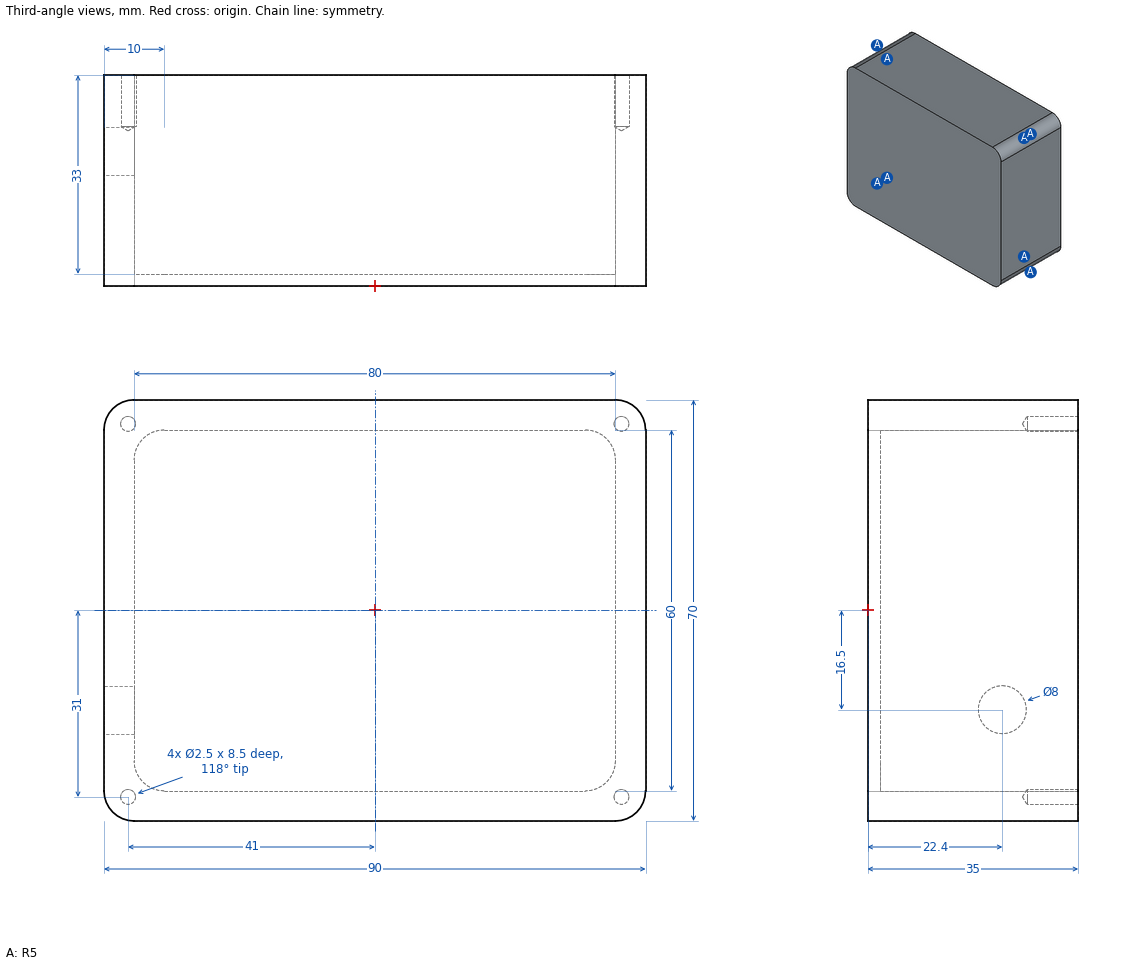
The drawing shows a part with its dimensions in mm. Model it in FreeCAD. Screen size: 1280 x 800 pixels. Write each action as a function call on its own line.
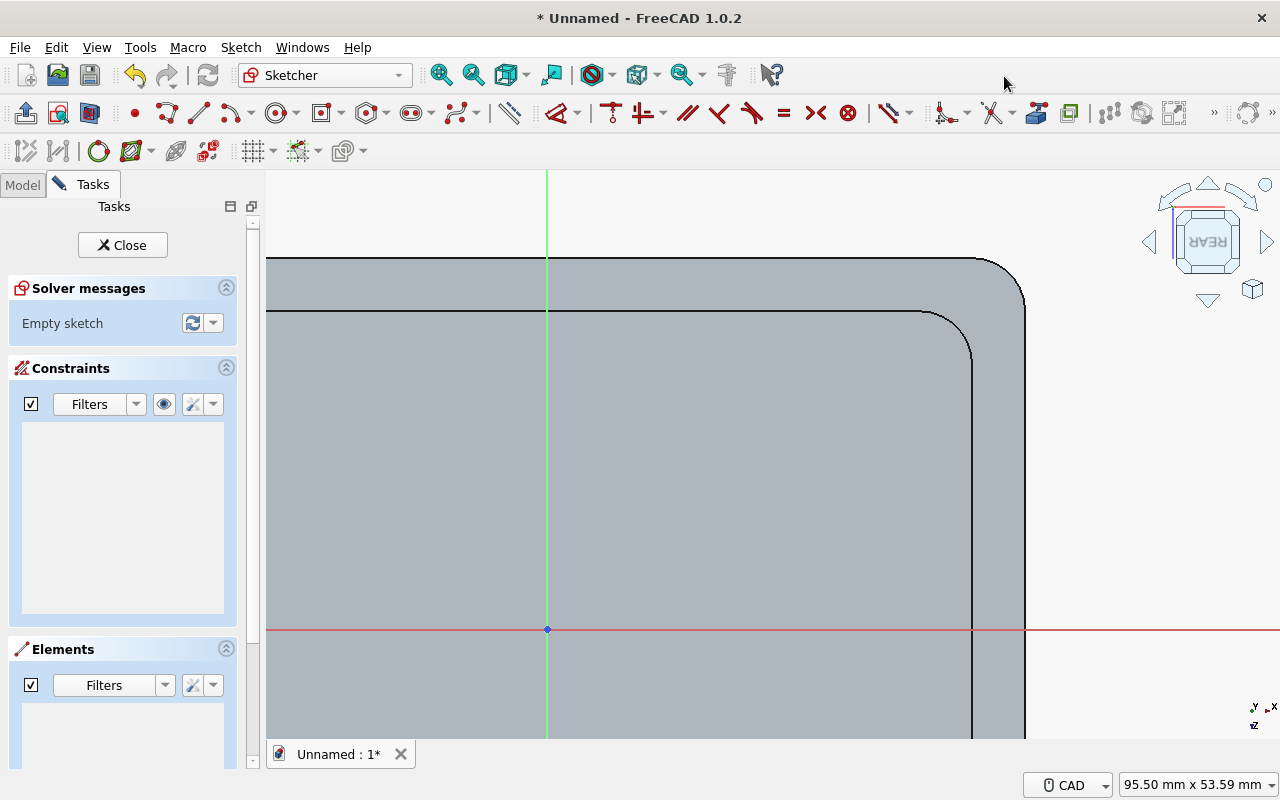
scroll(896, 241, down, 3)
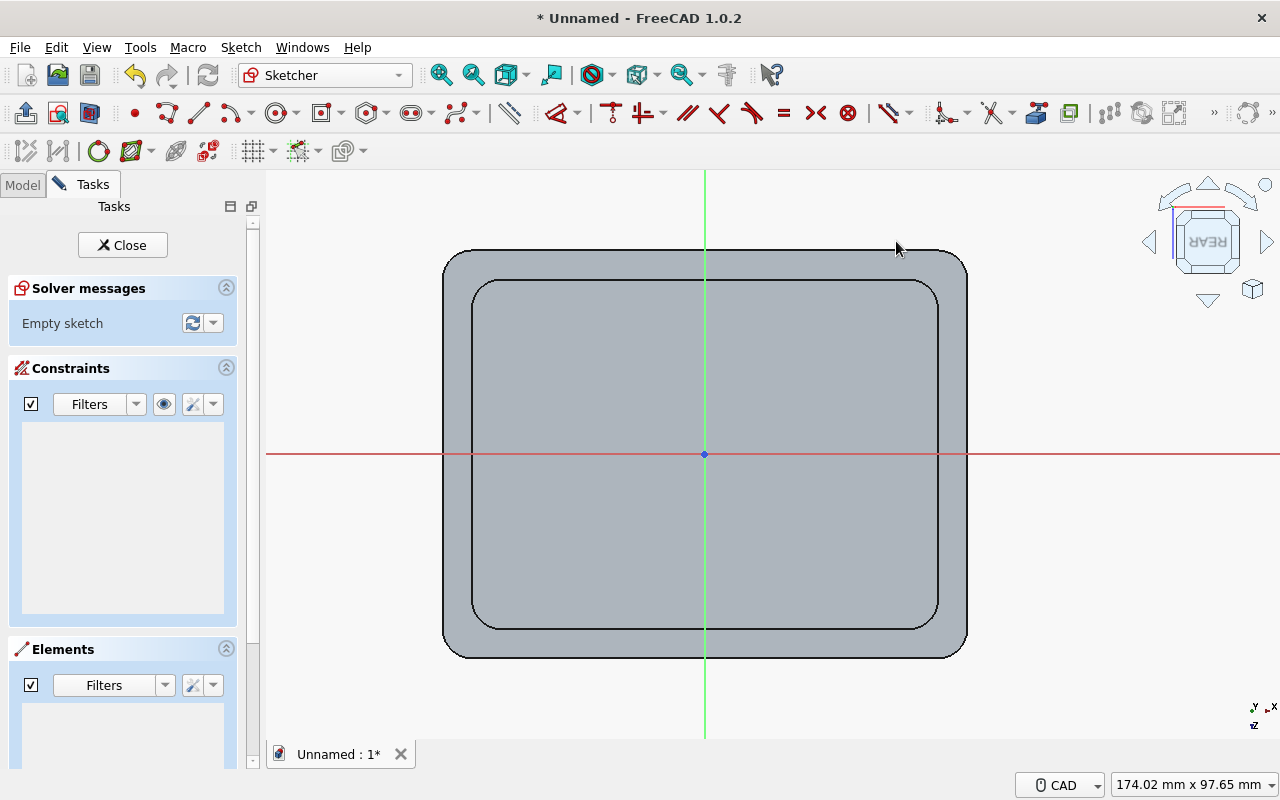
click(276, 114)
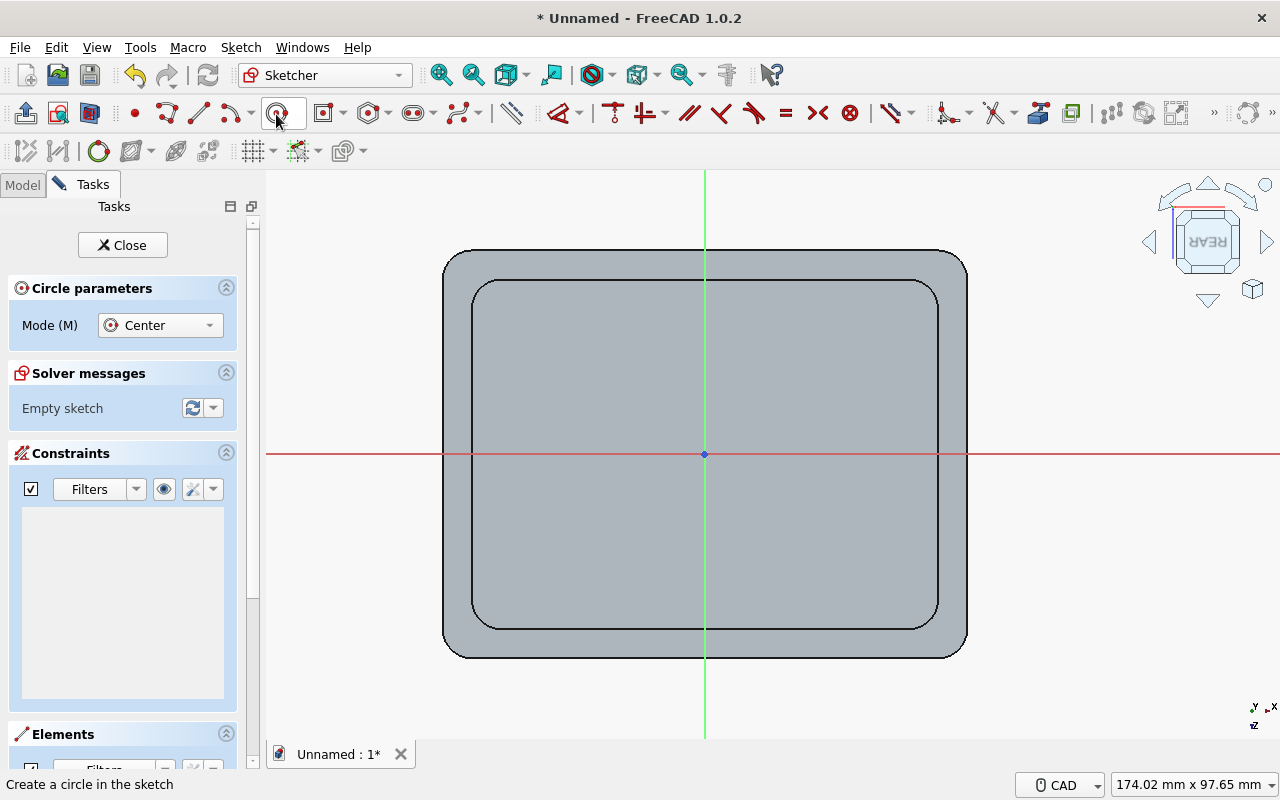
scroll(466, 274, up, 6)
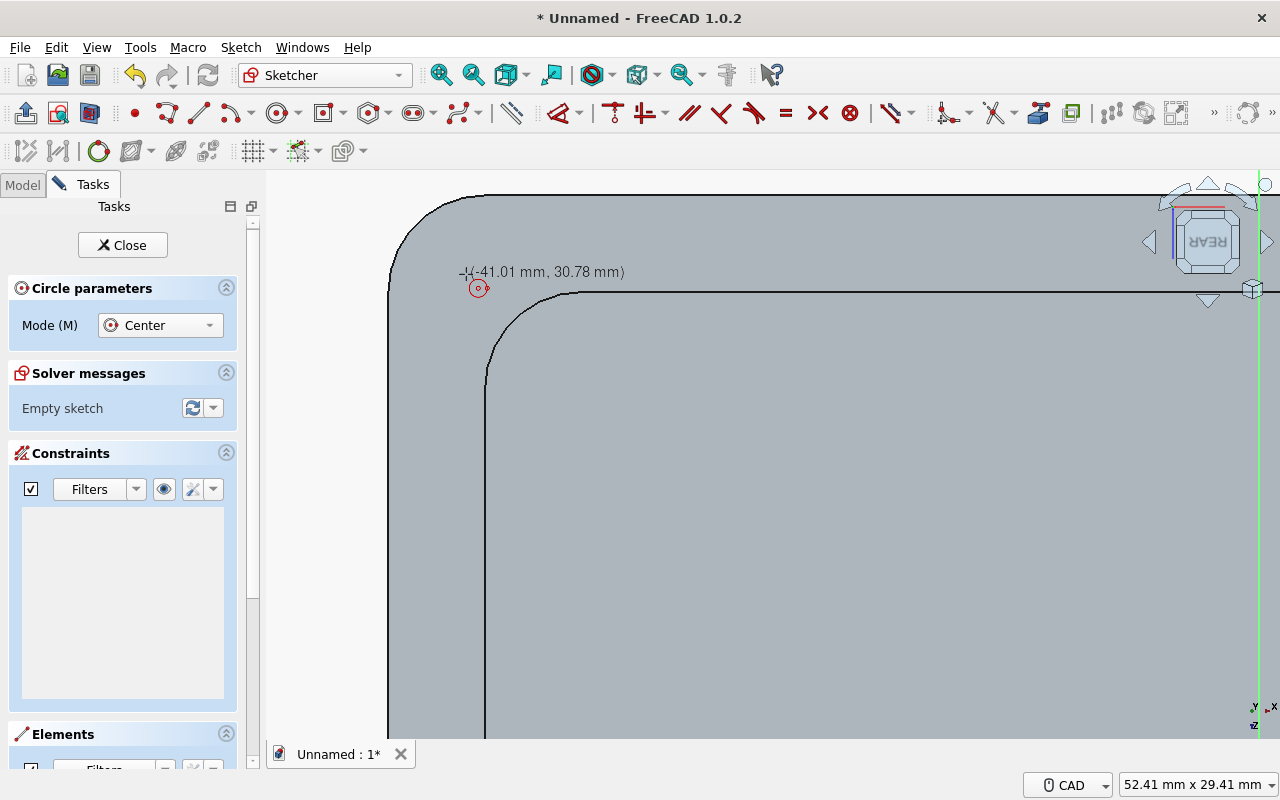
click(466, 273)
click(483, 256)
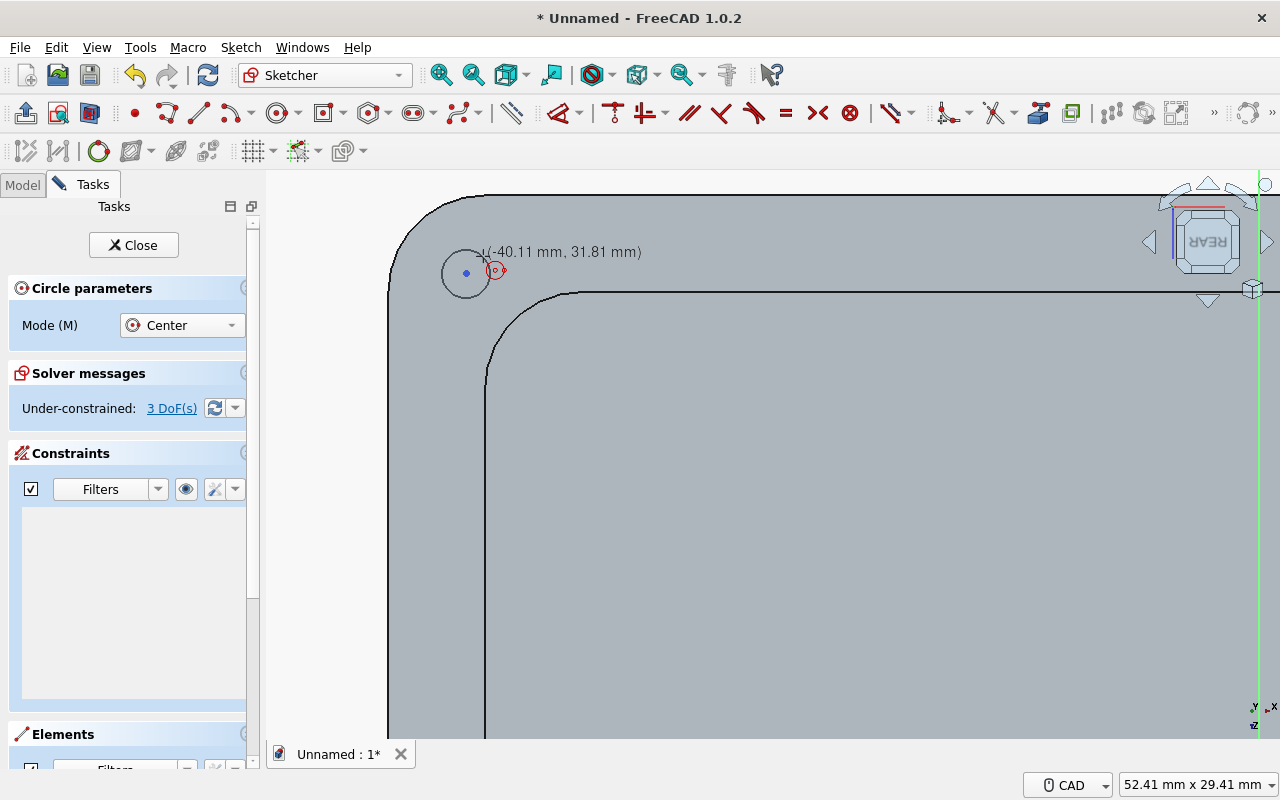
scroll(466, 274, down, 6)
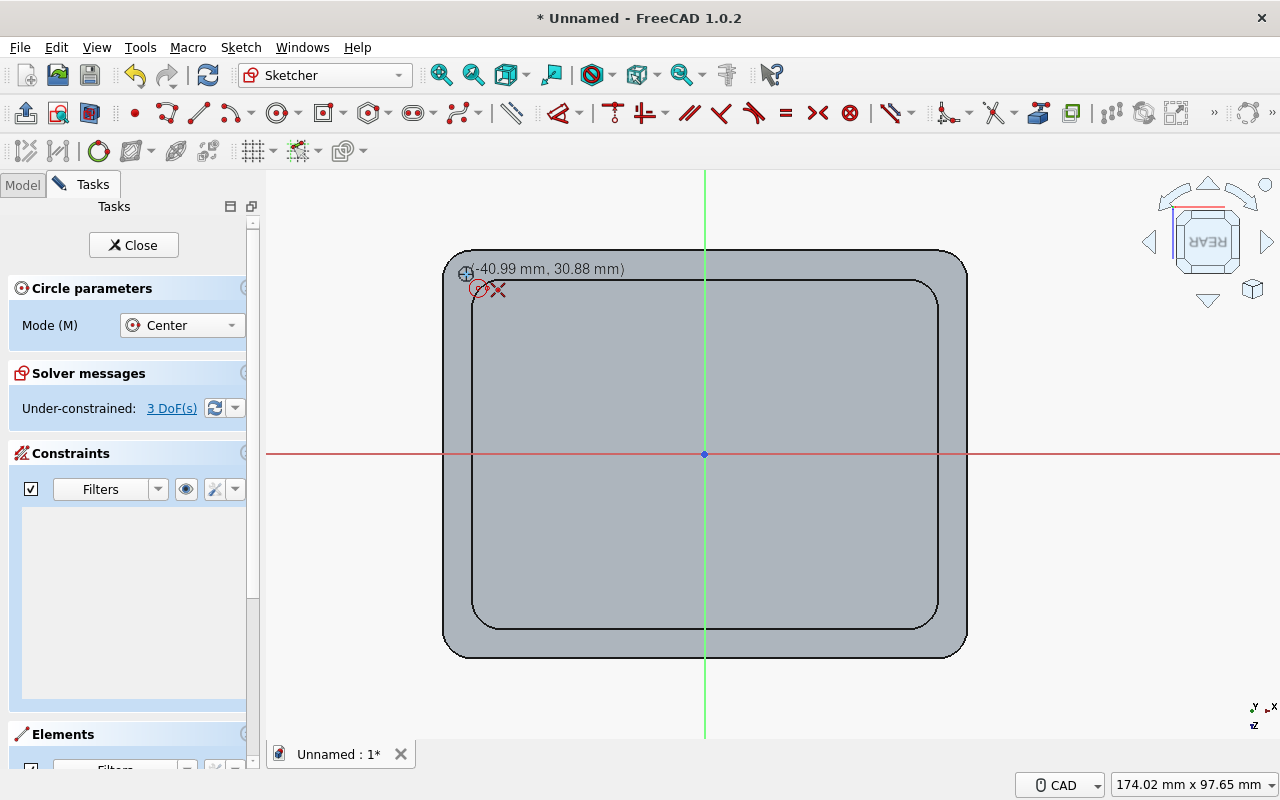
scroll(944, 274, up, 6)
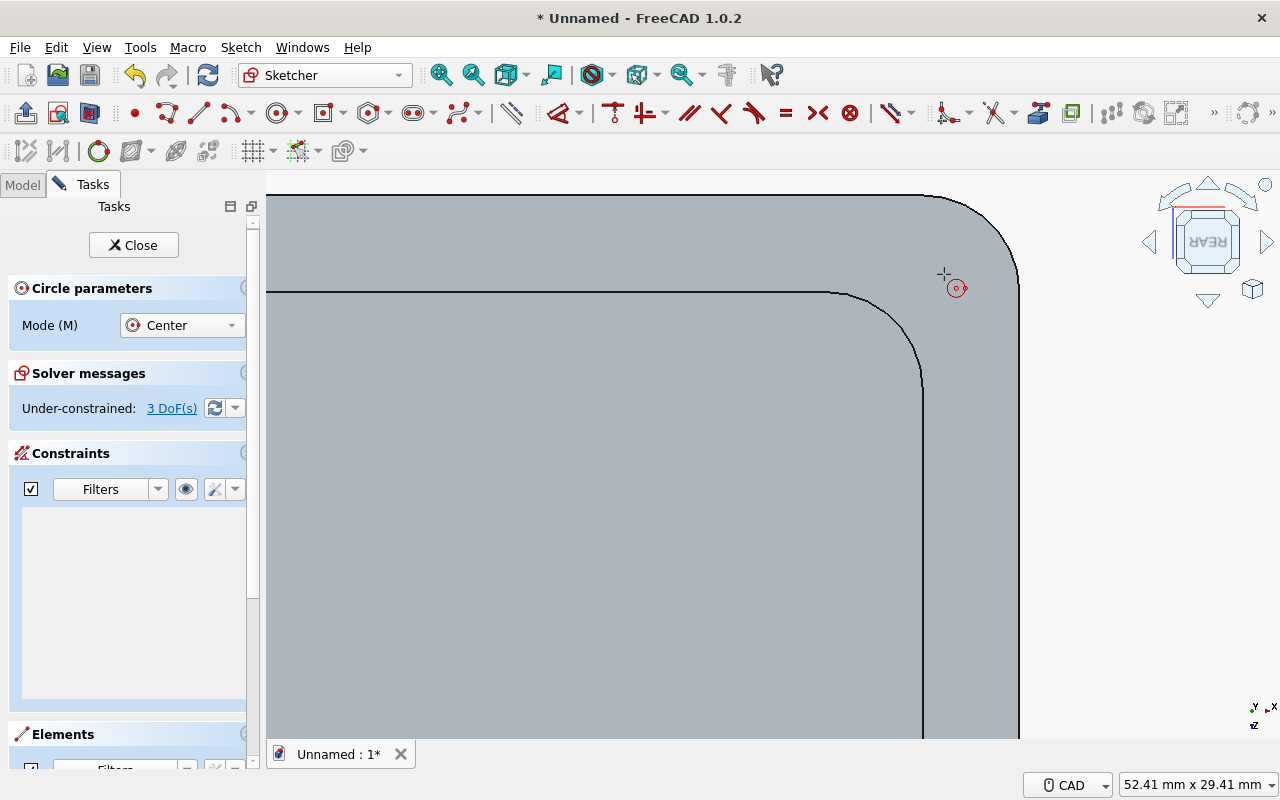
click(942, 273)
click(959, 256)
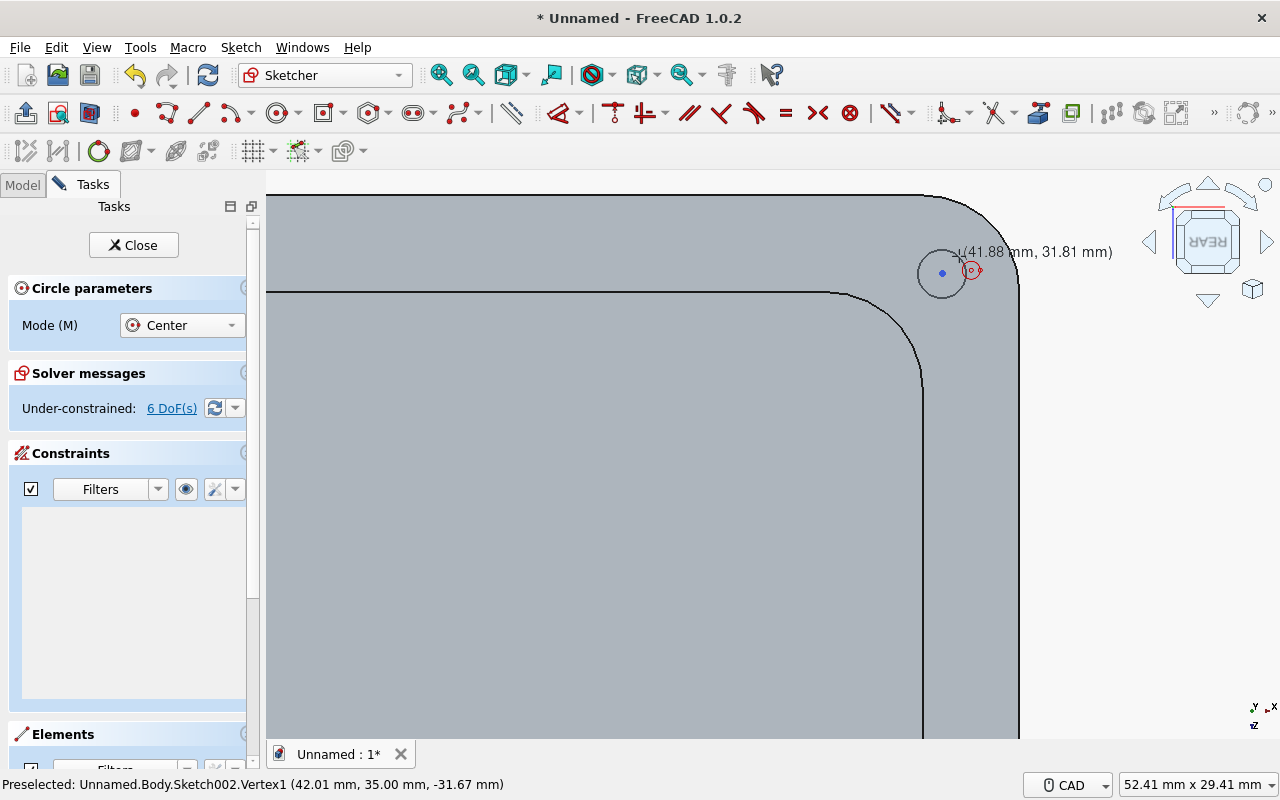
scroll(944, 274, down, 6)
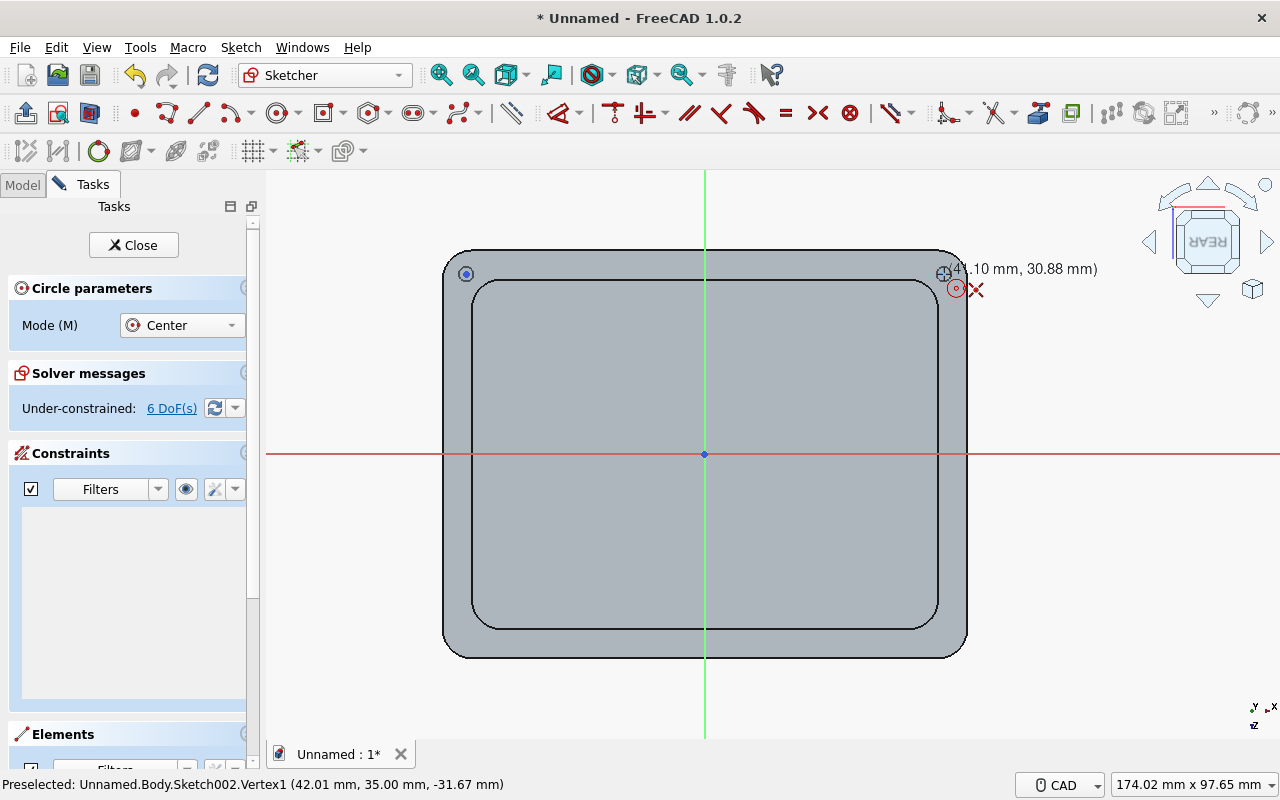
scroll(944, 635, up, 6)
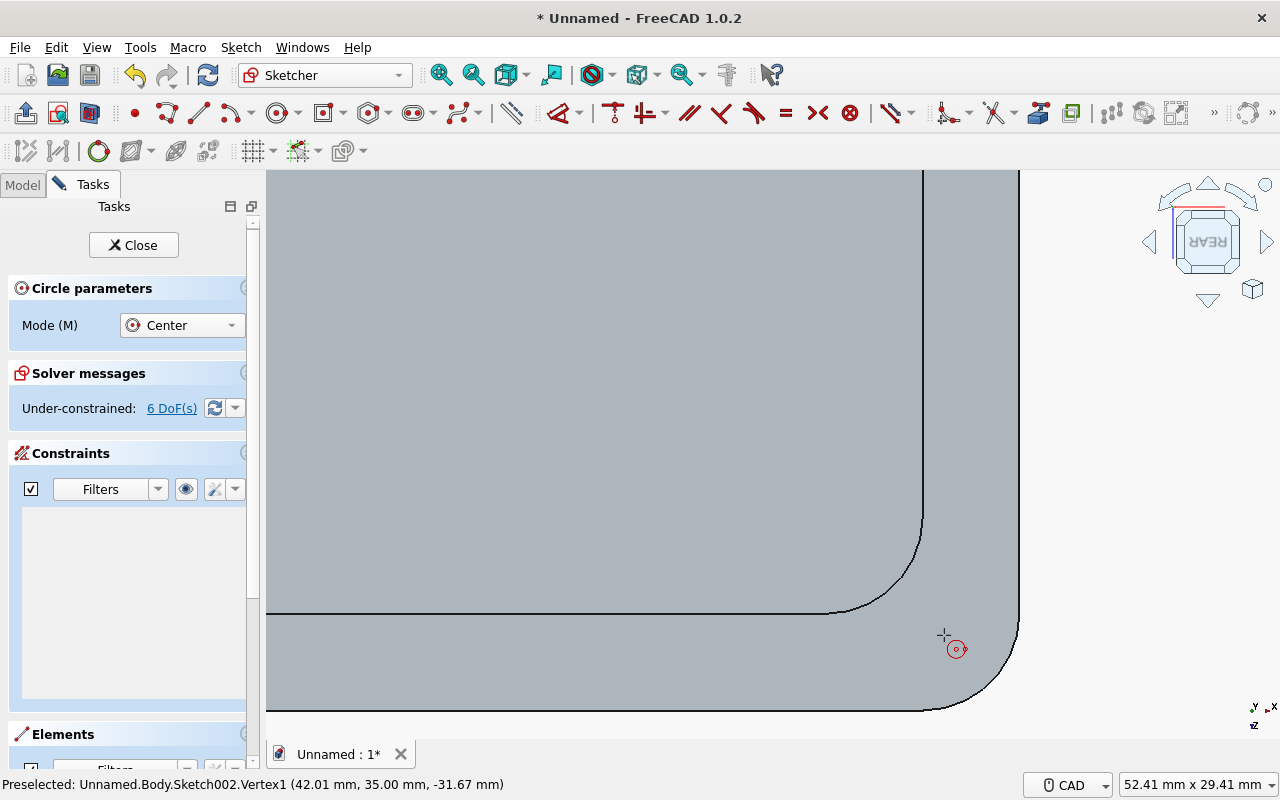
click(942, 633)
click(959, 616)